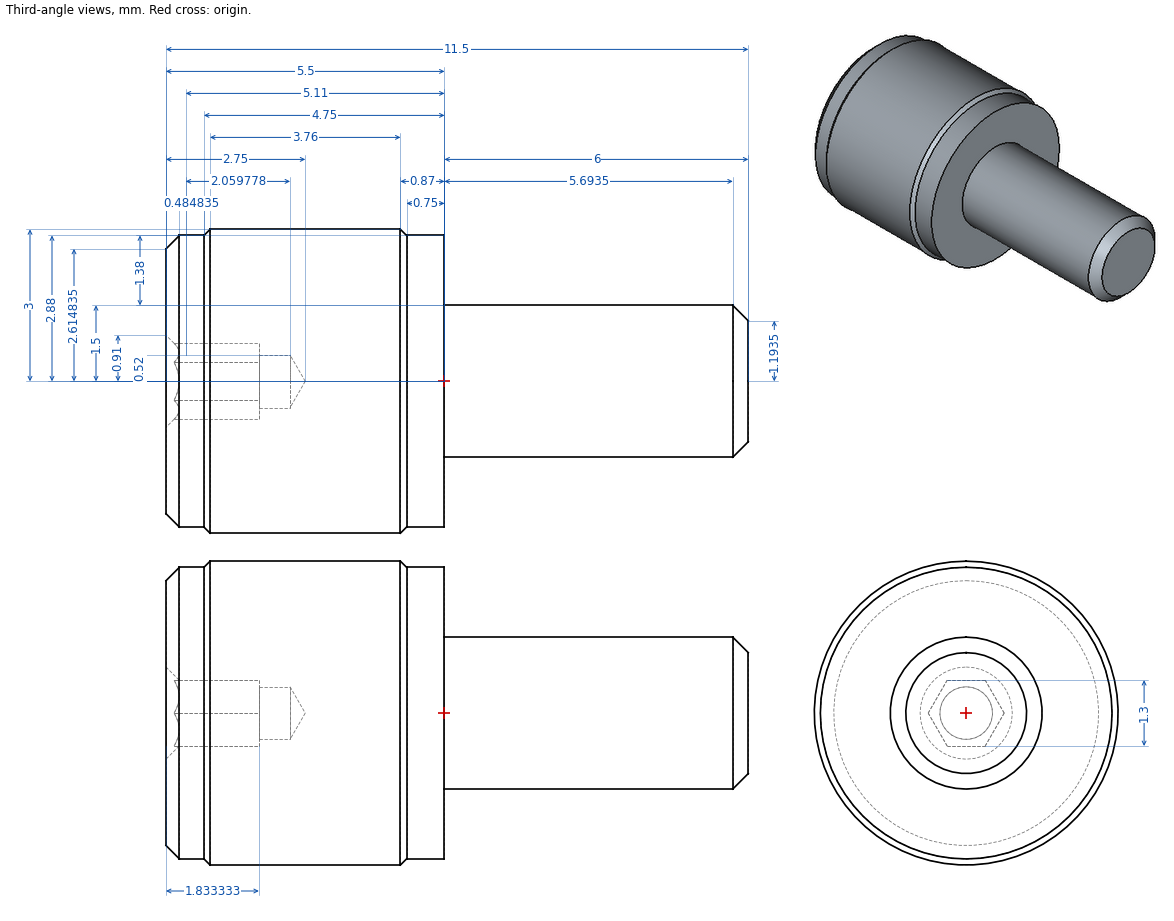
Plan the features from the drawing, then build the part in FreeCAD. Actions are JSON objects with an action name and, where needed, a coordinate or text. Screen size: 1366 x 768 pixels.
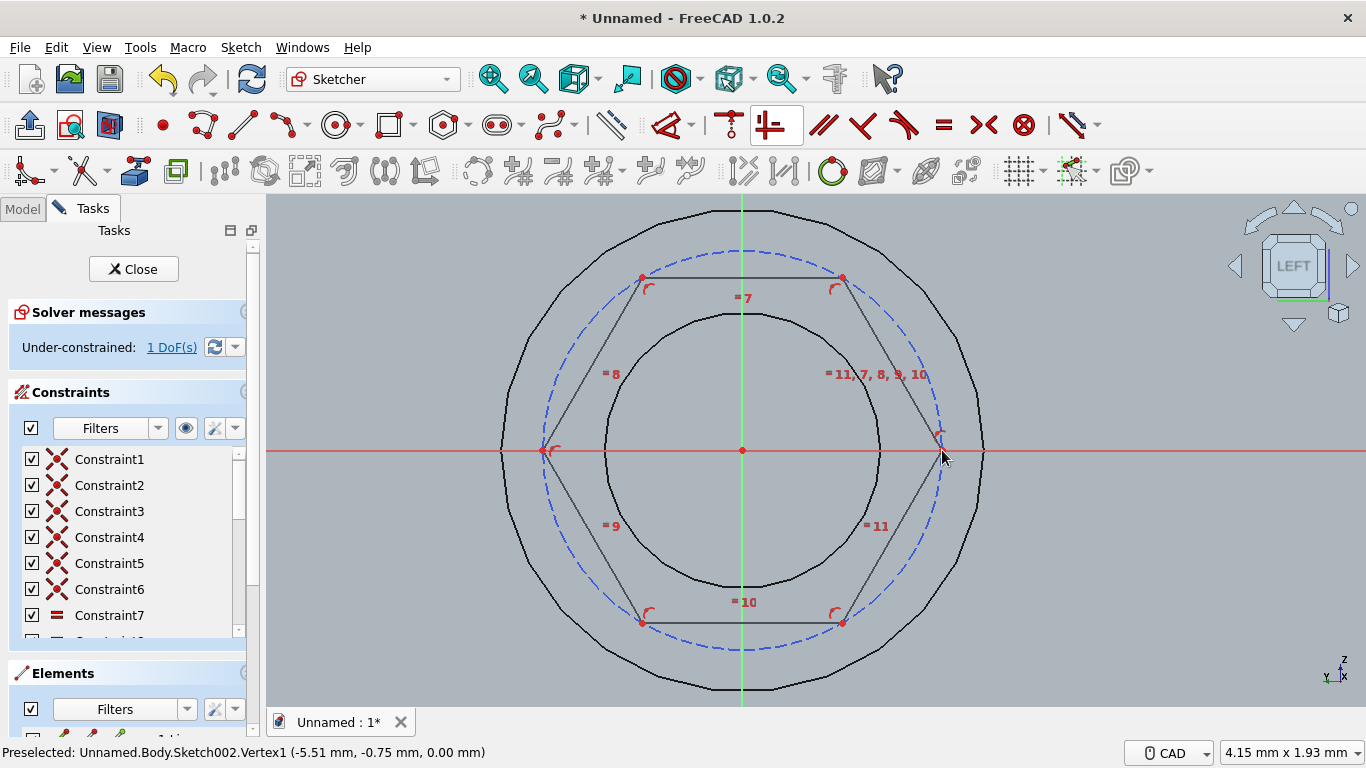
{"action": "left_click", "coordinate": [666, 126]}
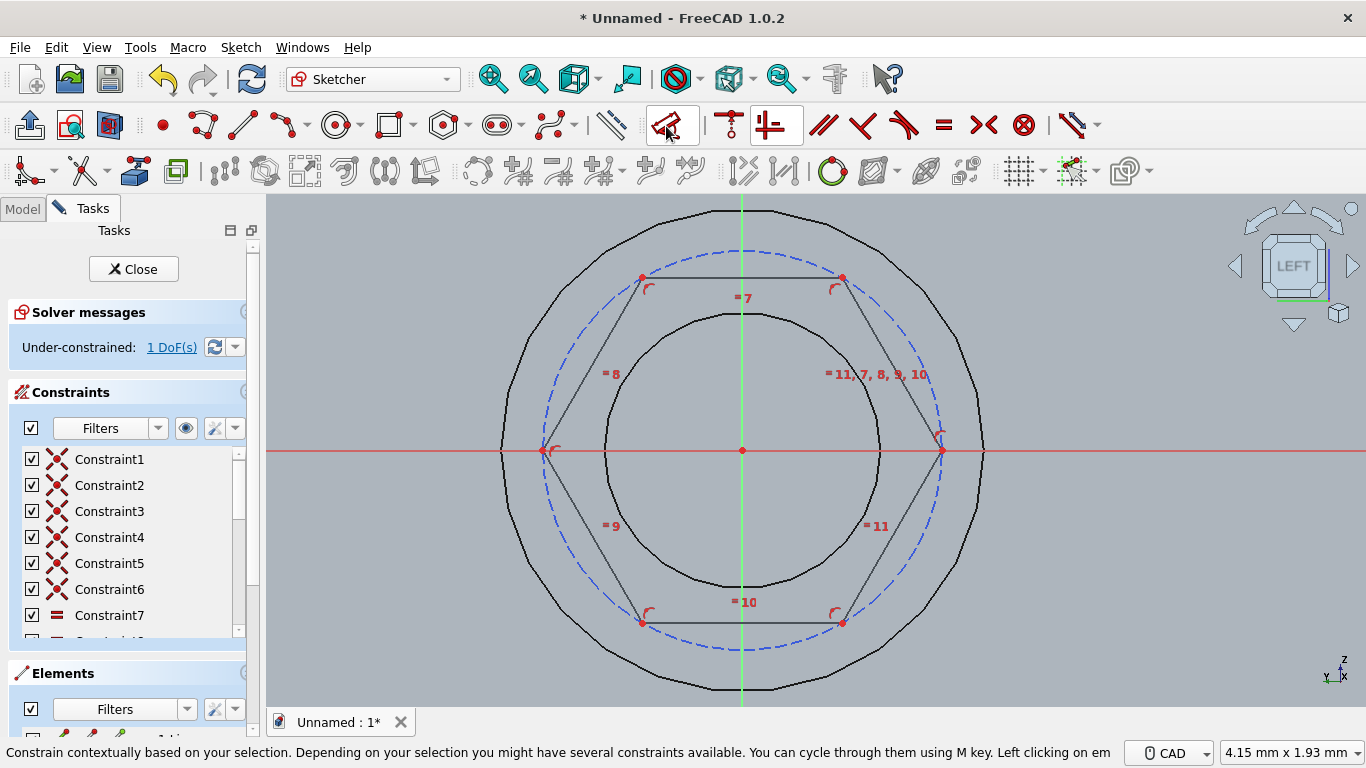
{"action": "left_click", "coordinate": [643, 623]}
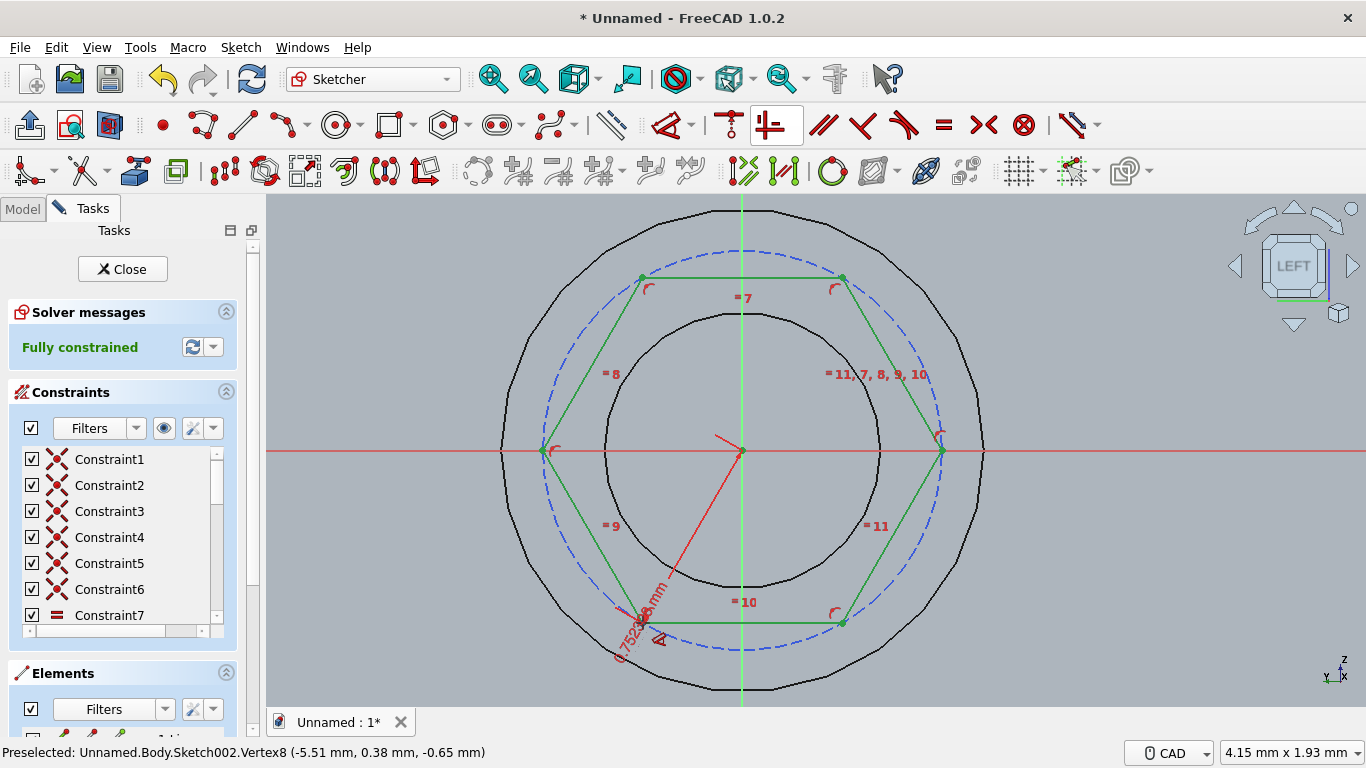
{"action": "left_click", "coordinate": [842, 278]}
{"action": "left_click", "coordinate": [876, 371]}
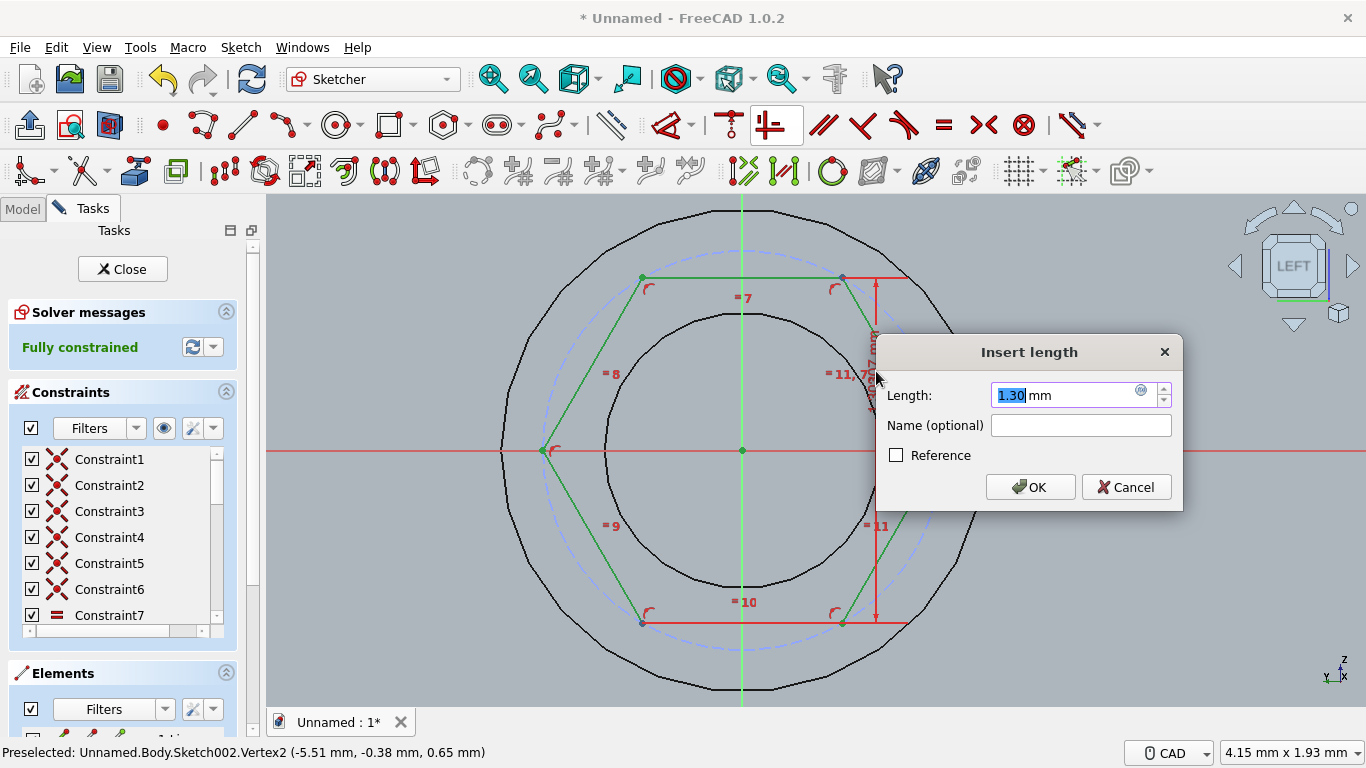
{"action": "type", "text": "1.3"}
{"action": "key", "text": "Return"}
{"action": "key", "text": "Escape"}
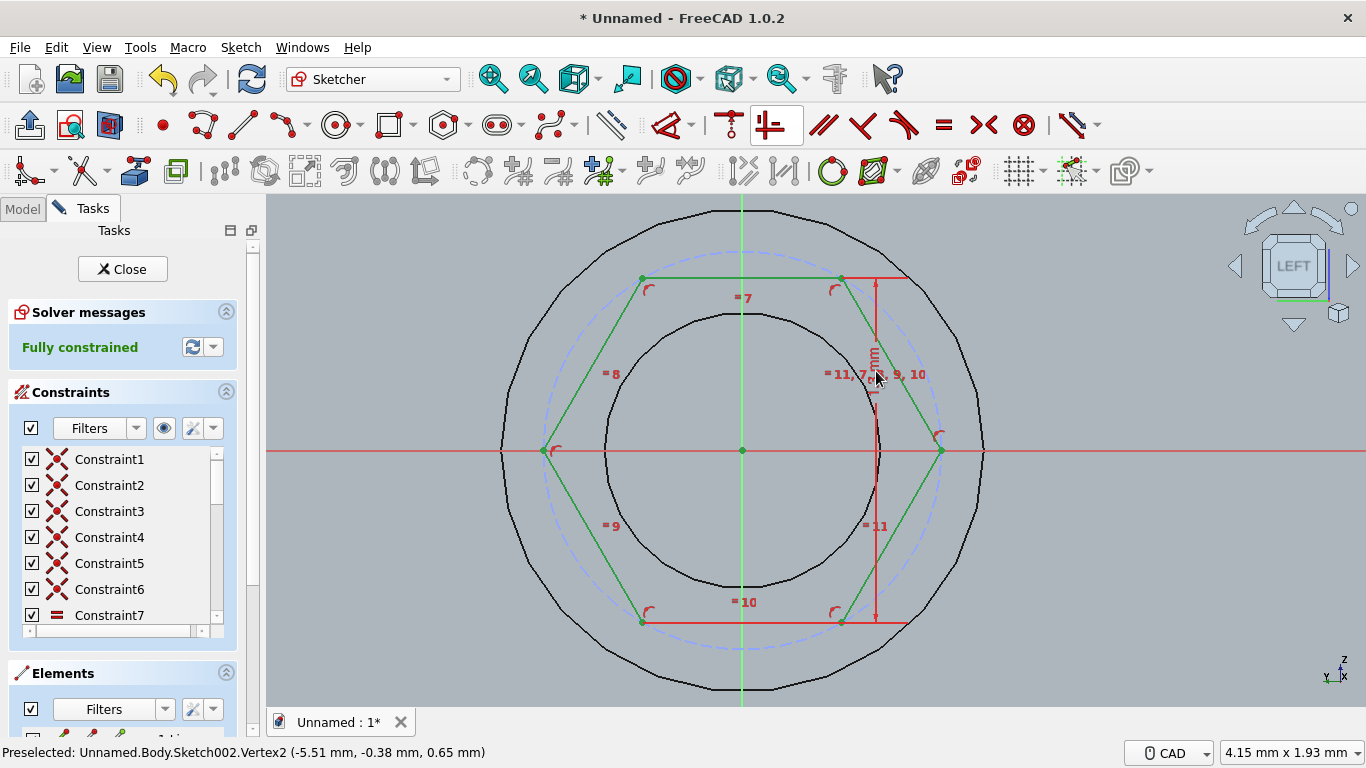
{"action": "left_click", "coordinate": [123, 269]}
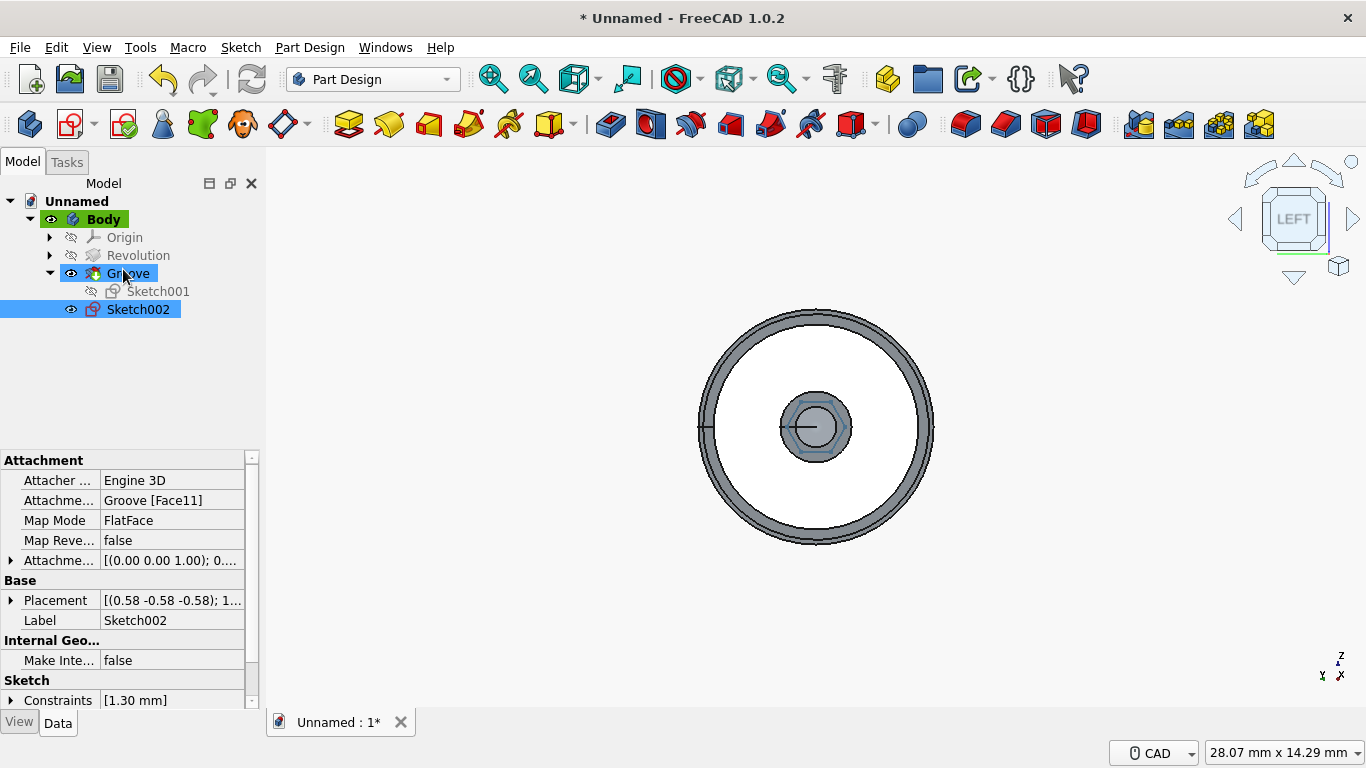
{"action": "left_click", "coordinate": [612, 124]}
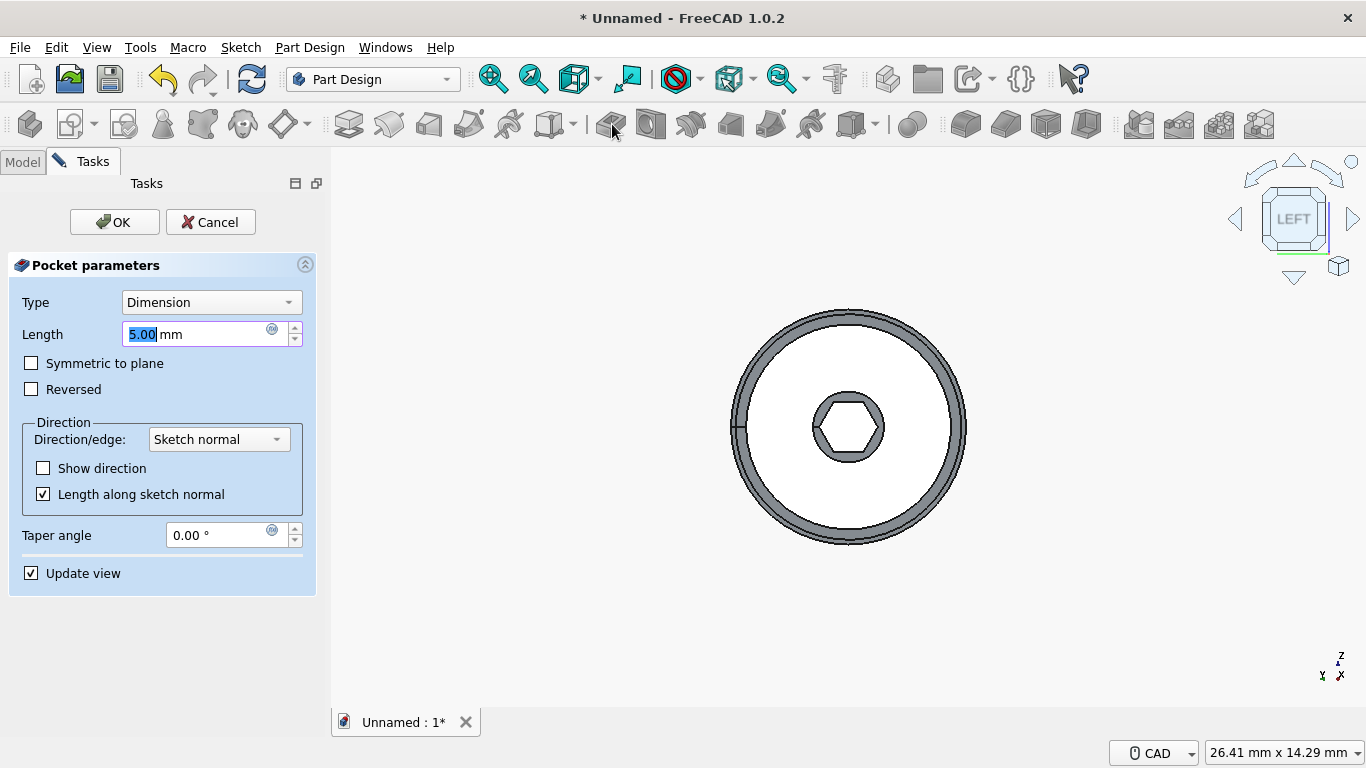
{"action": "type", "text": "1.833333"}
{"action": "key", "text": "Tab"}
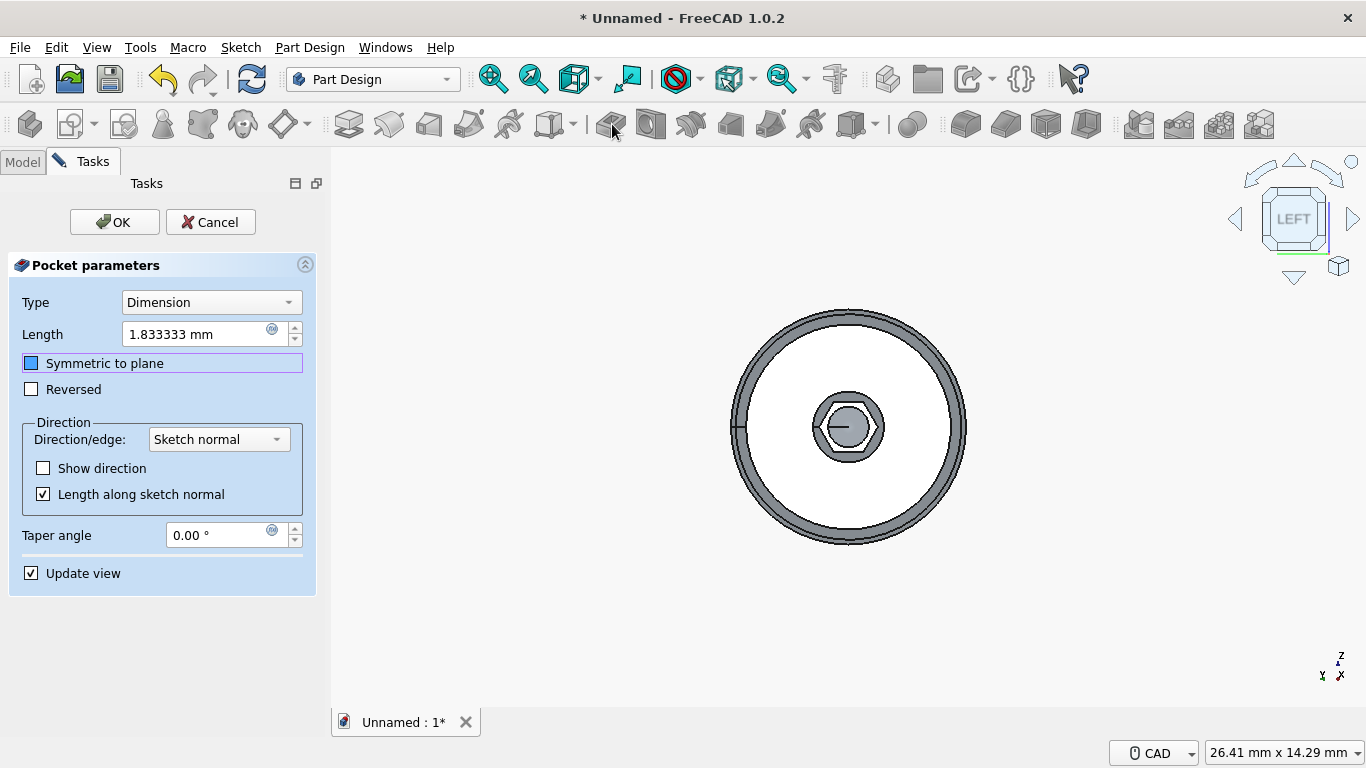
{"action": "left_click", "coordinate": [115, 222]}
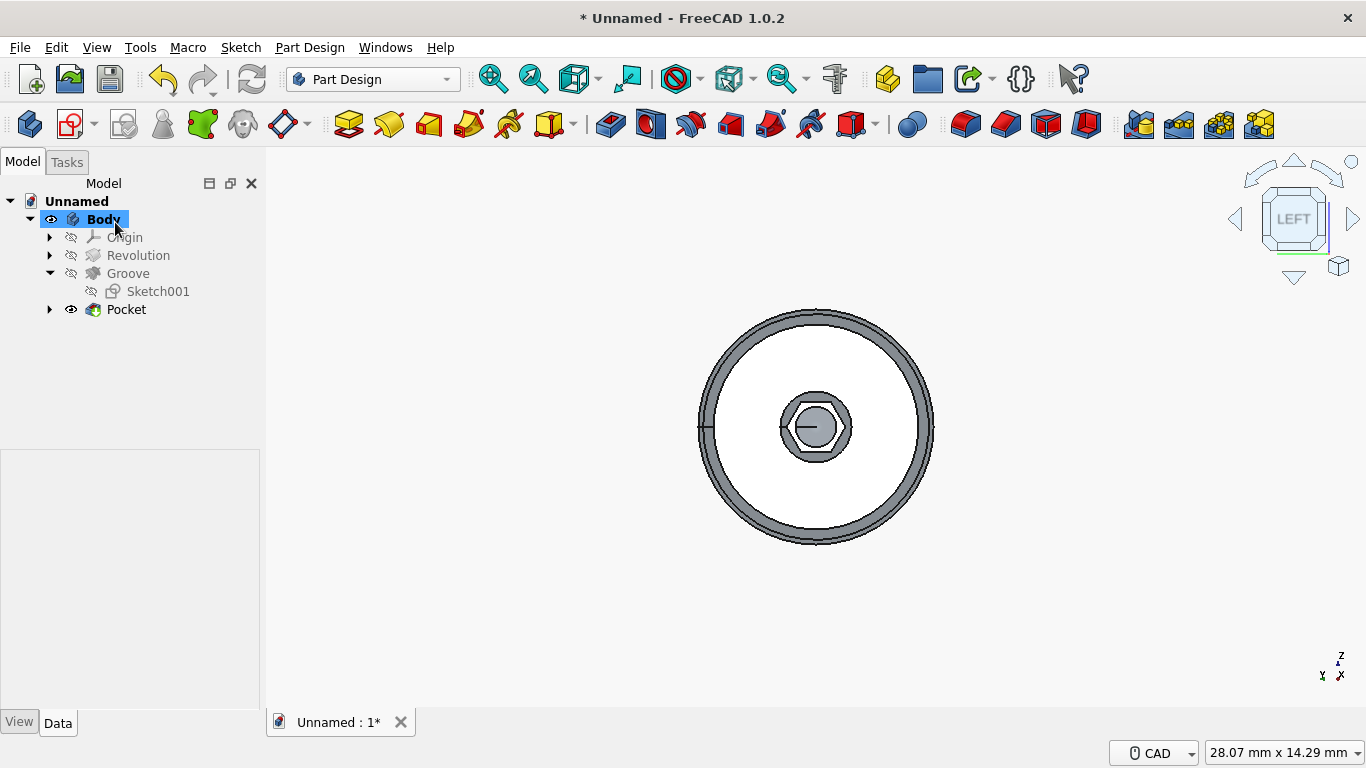
{"action": "key", "text": "0"}